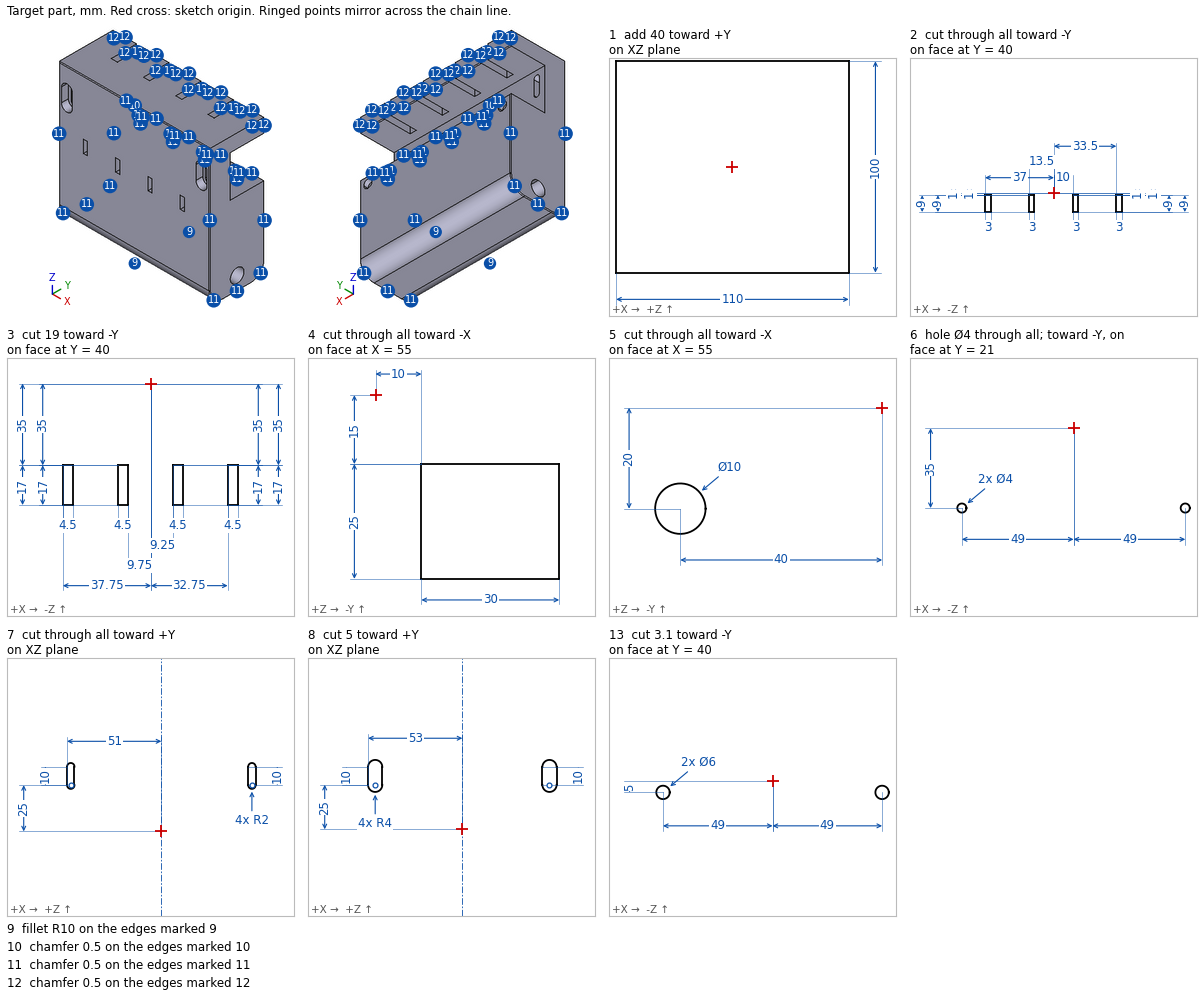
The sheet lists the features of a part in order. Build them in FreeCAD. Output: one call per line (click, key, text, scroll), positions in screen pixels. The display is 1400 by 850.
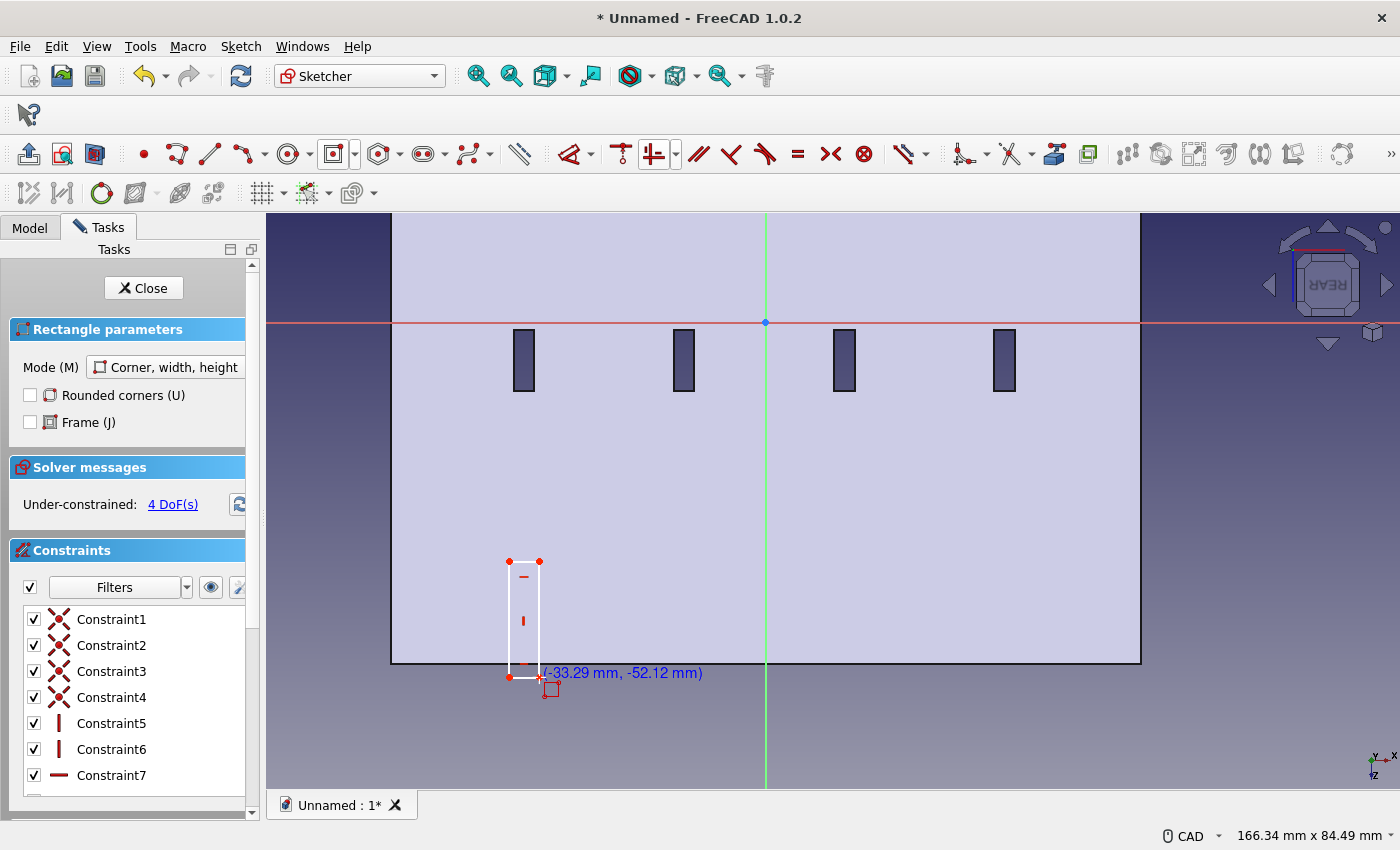
click(669, 561)
click(699, 677)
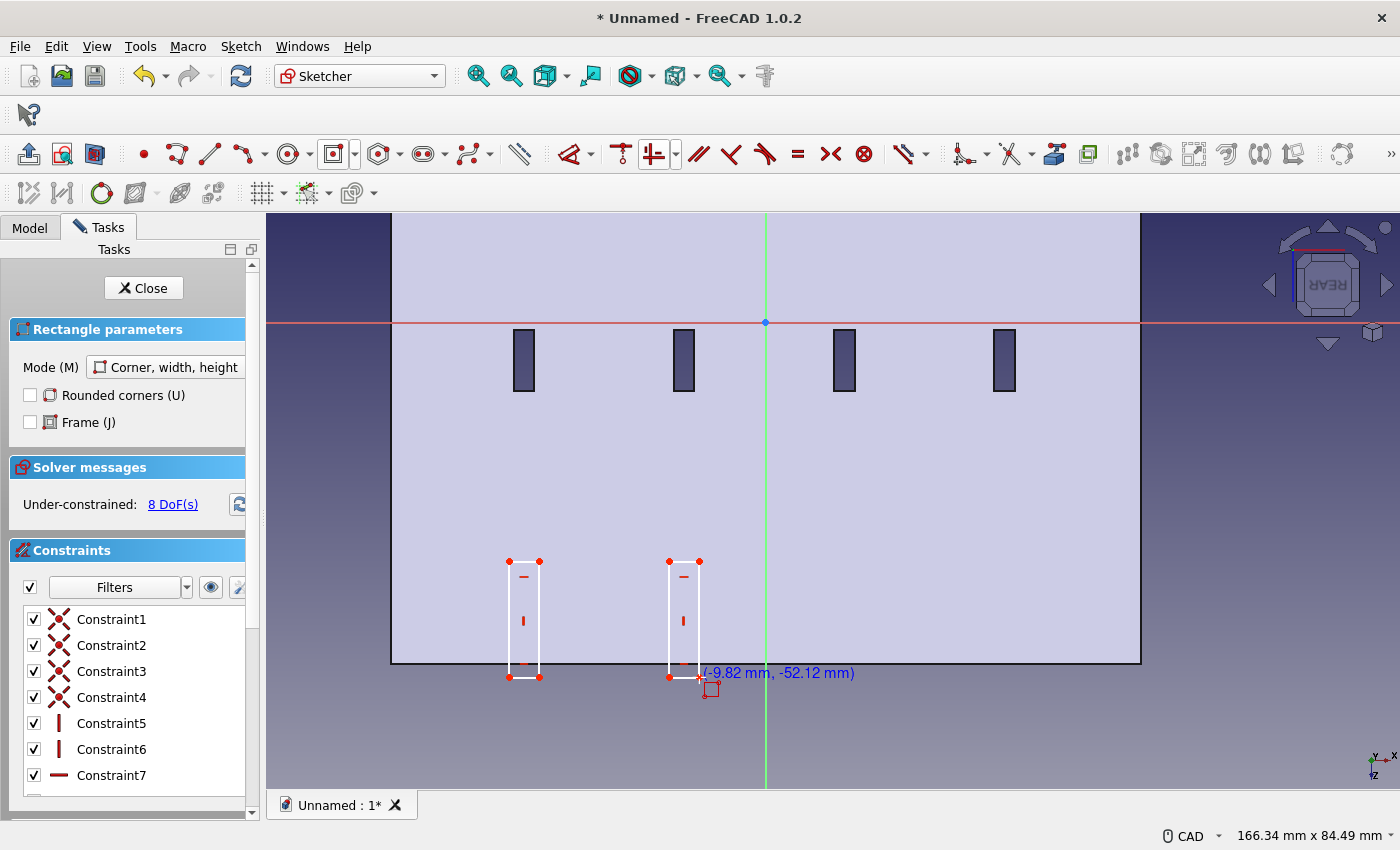
click(829, 561)
click(860, 677)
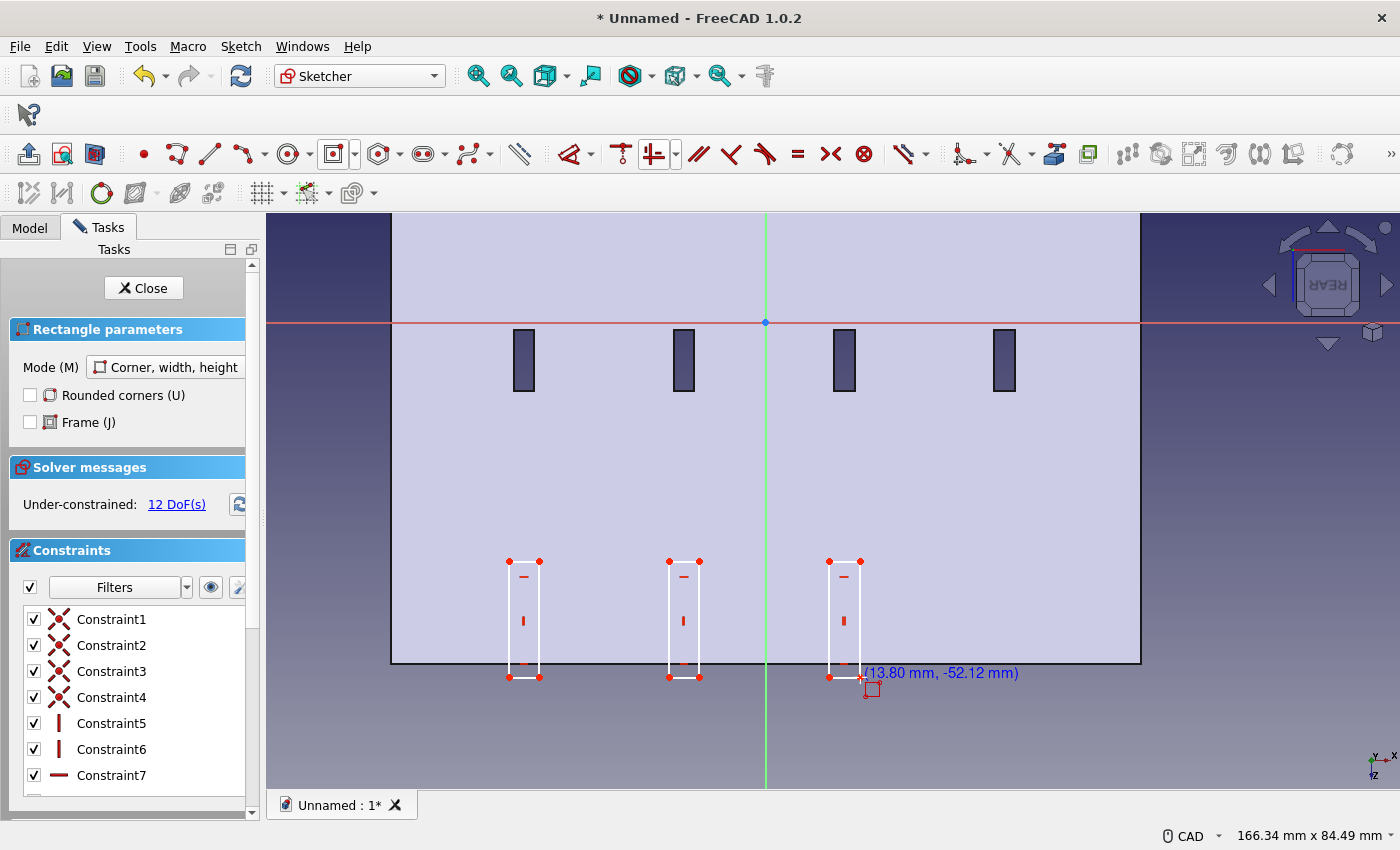
click(989, 561)
click(1020, 677)
key(Escape)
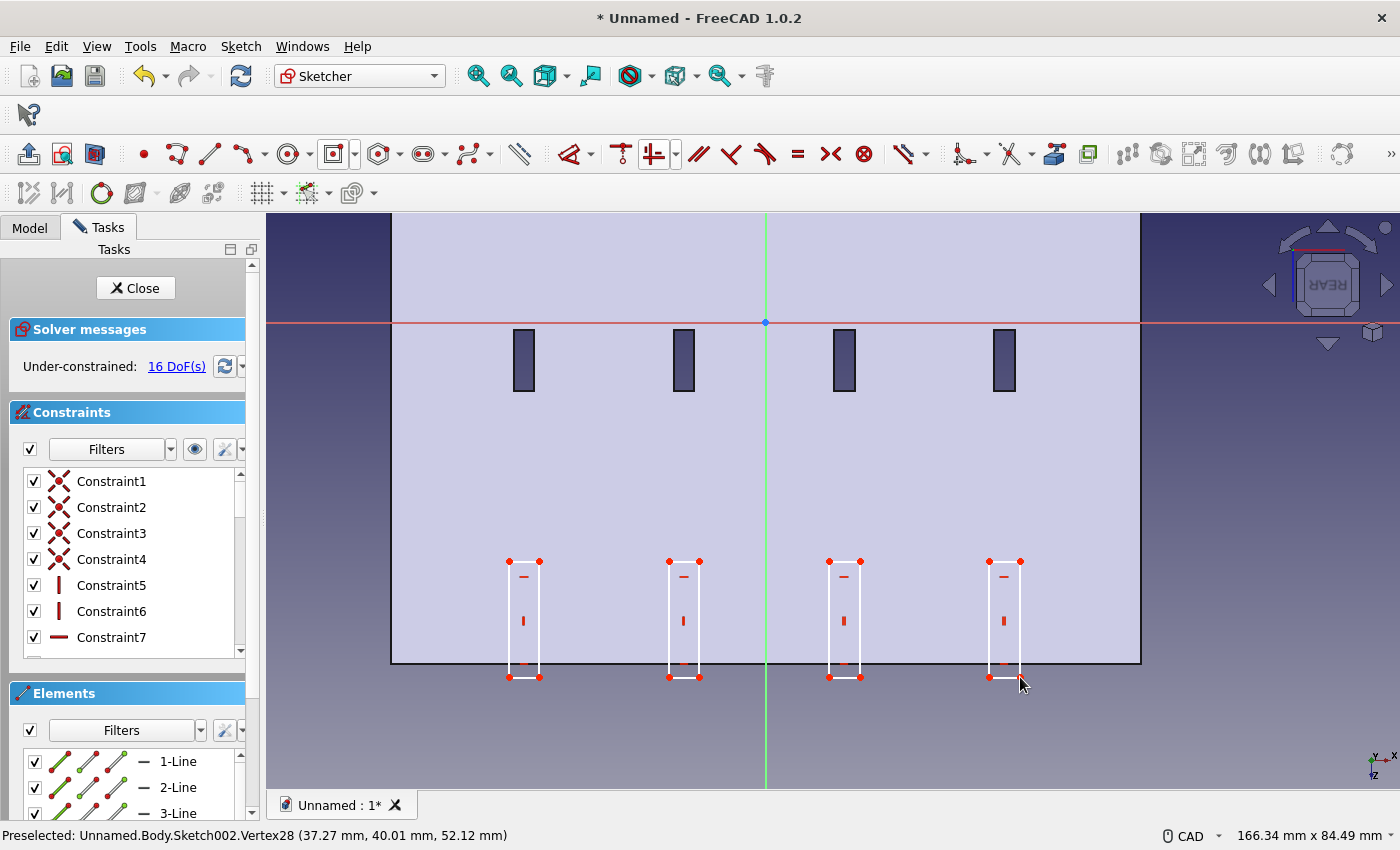
key(d)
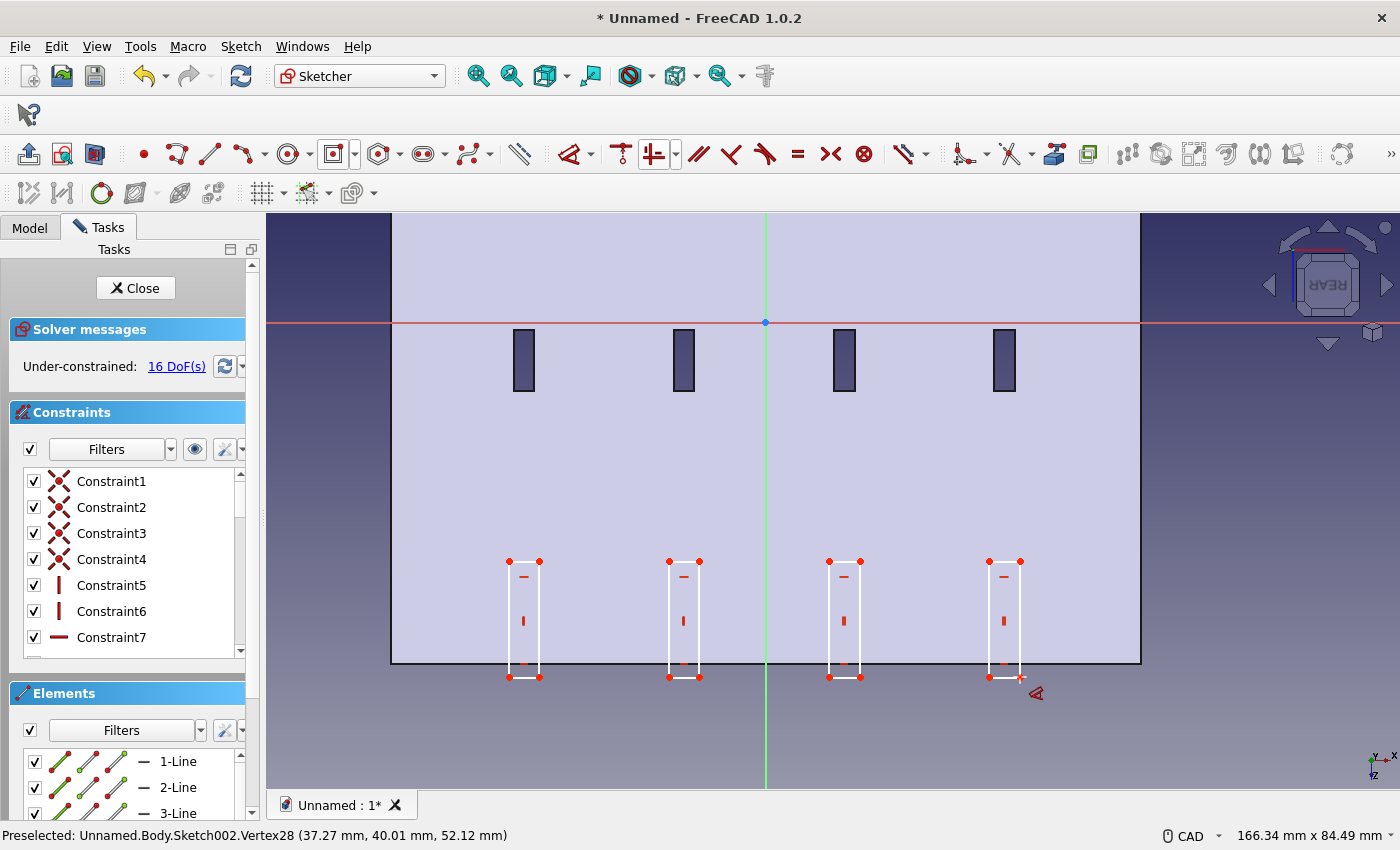
click(509, 597)
click(475, 620)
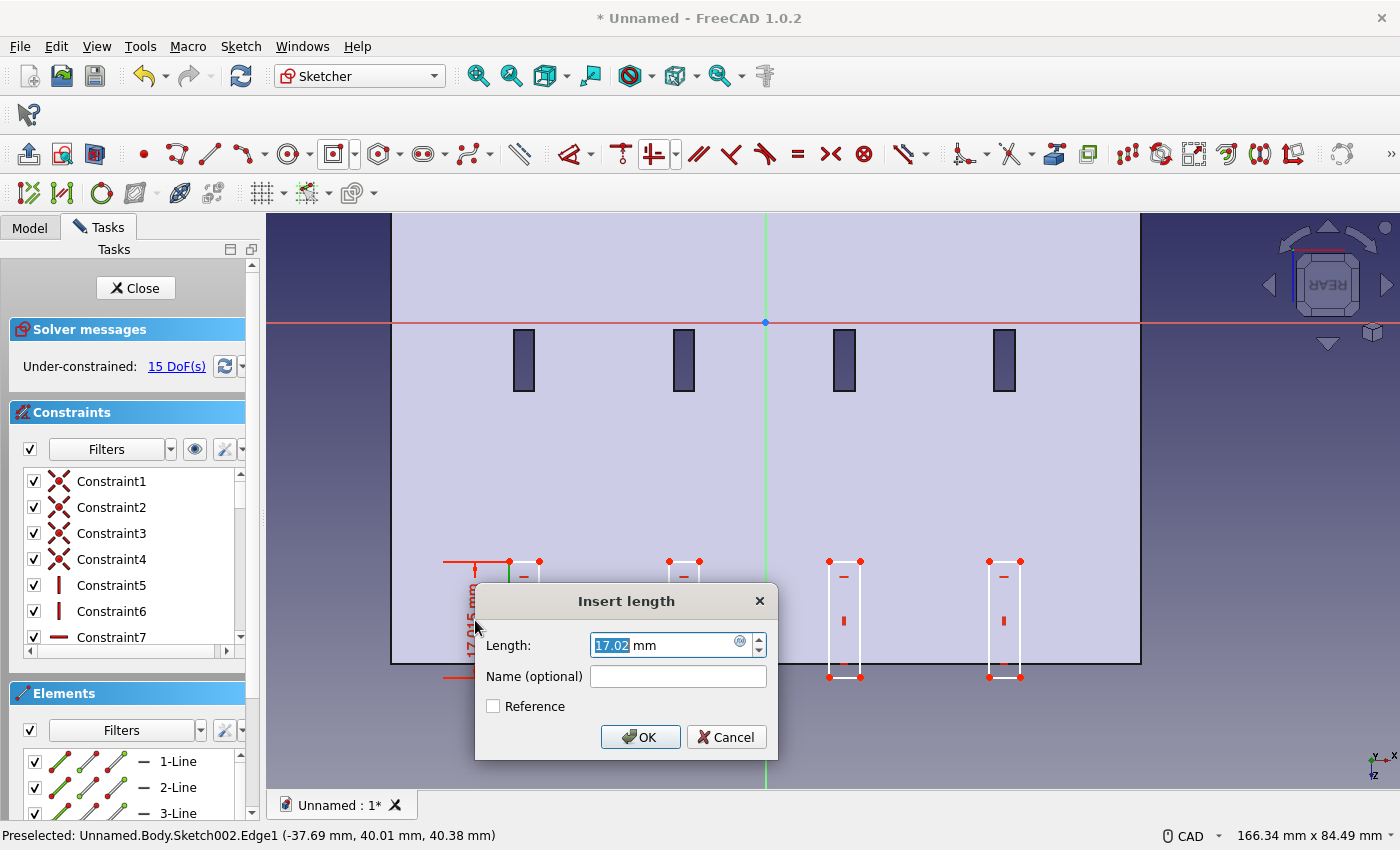
text(17)
key(Return)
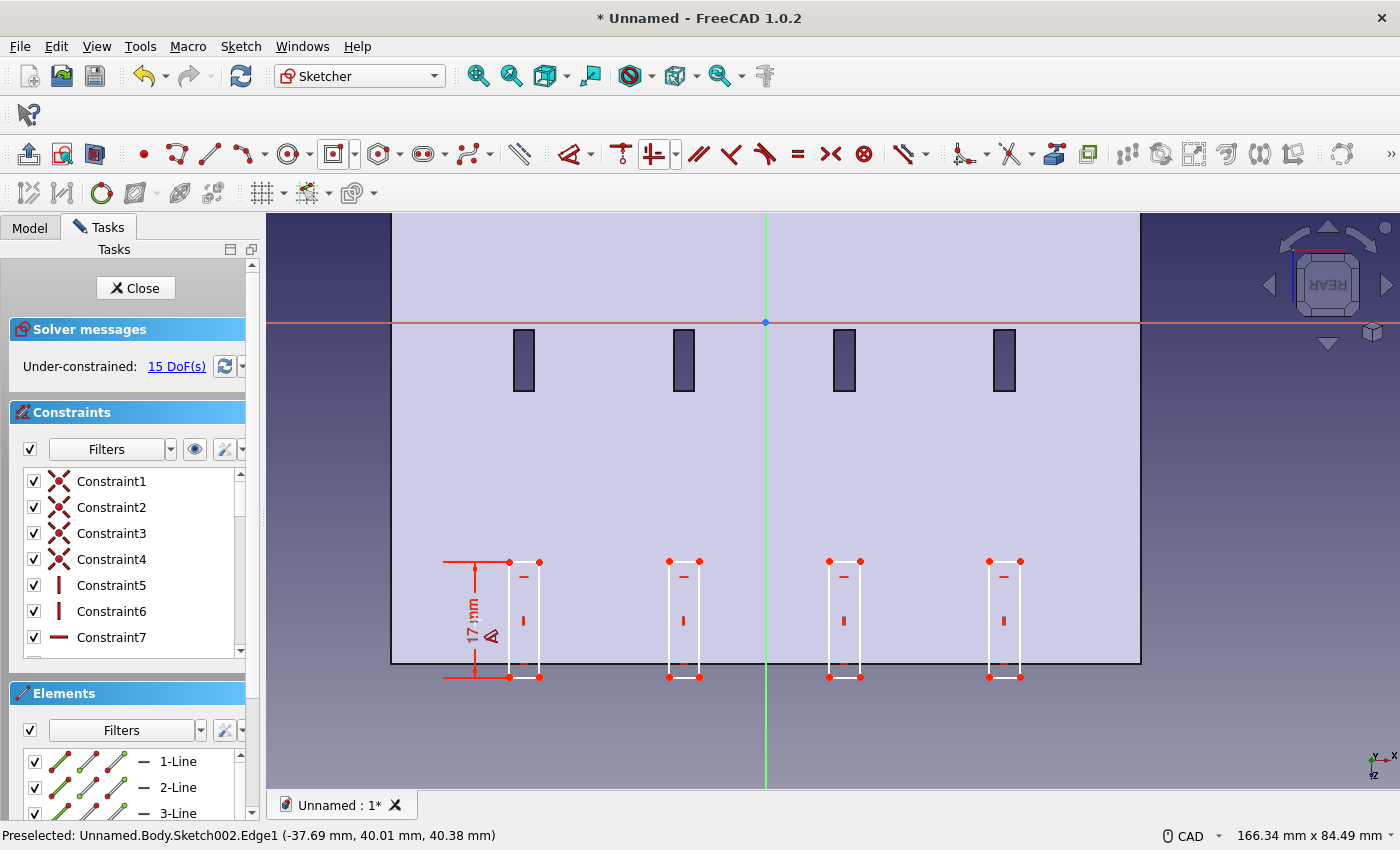
click(669, 597)
click(635, 620)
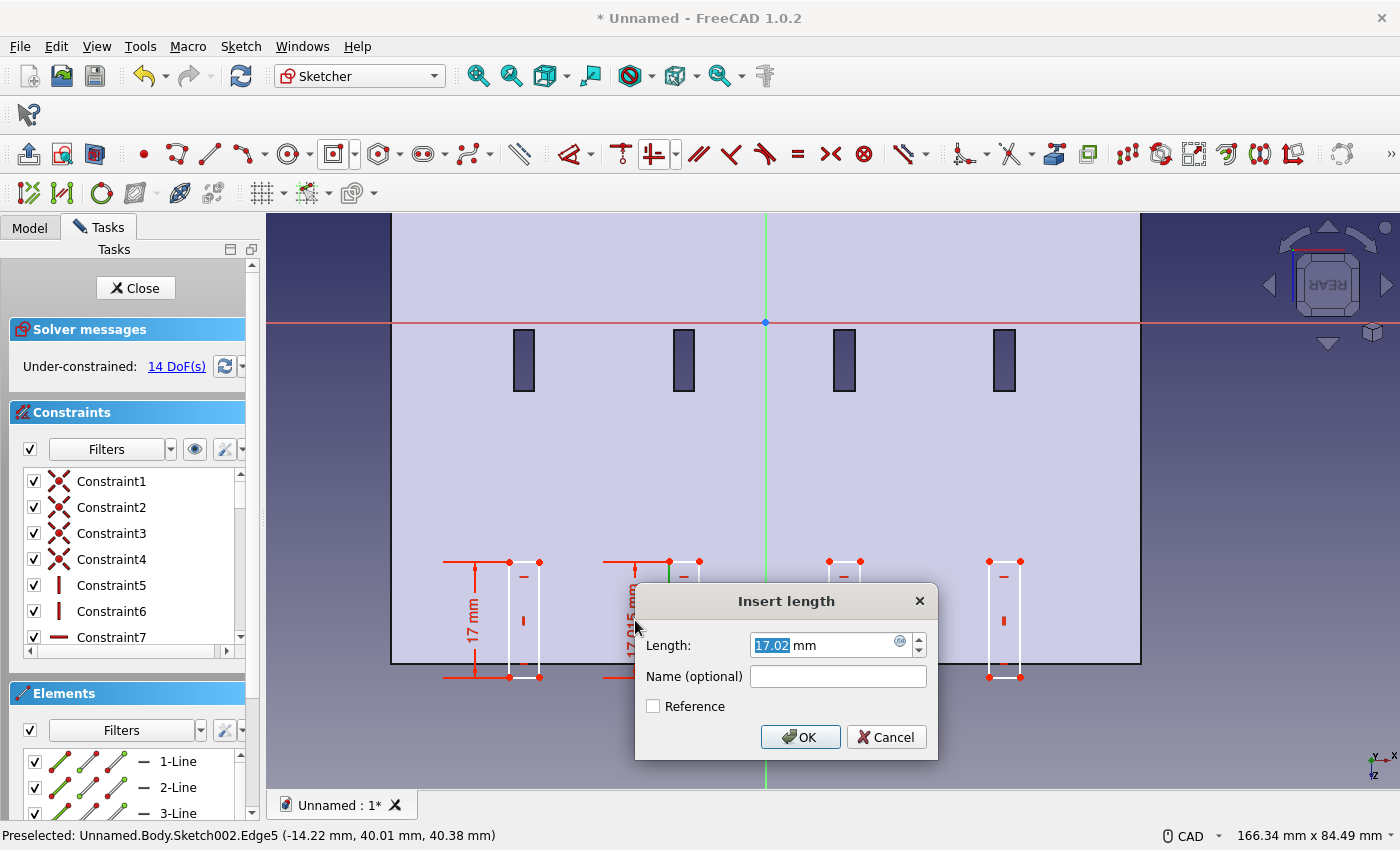
text(17)
key(Return)